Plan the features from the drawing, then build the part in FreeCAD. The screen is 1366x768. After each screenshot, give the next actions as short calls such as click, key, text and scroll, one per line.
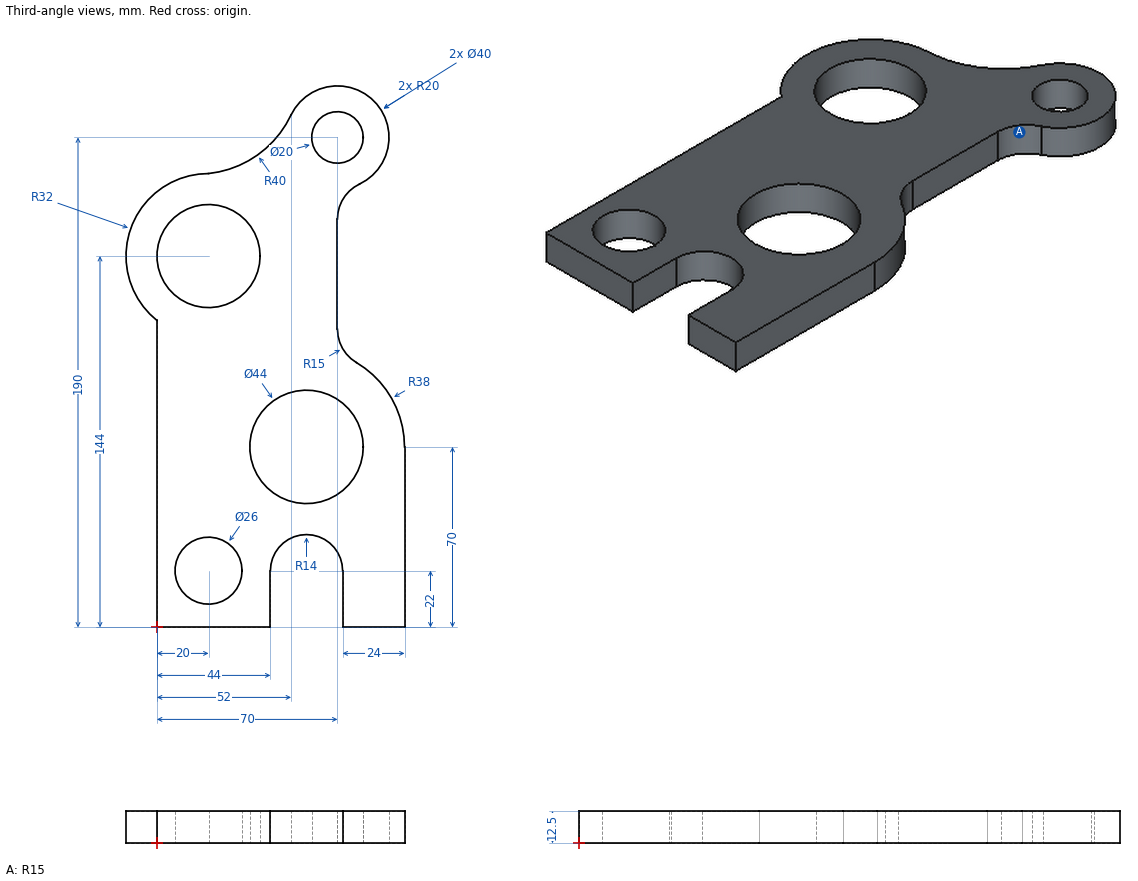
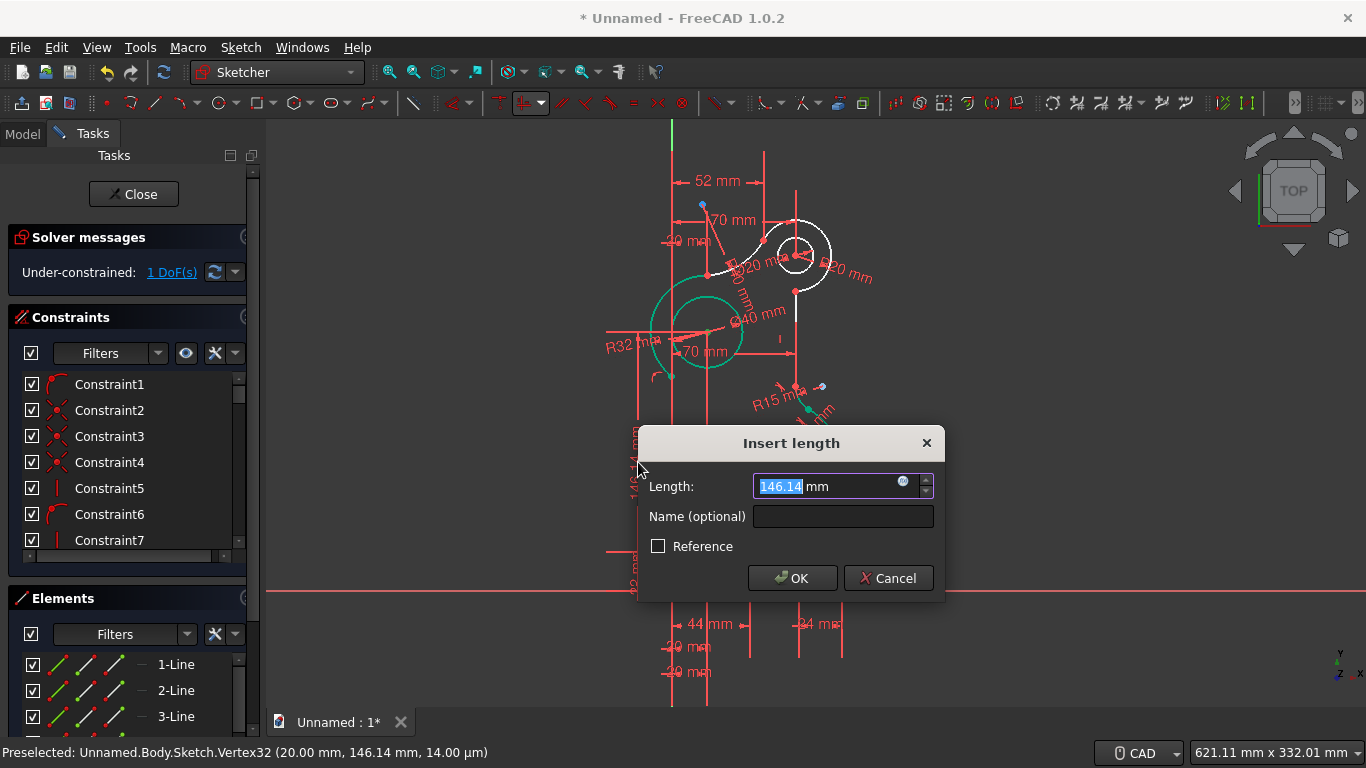
text(144)
key(Return)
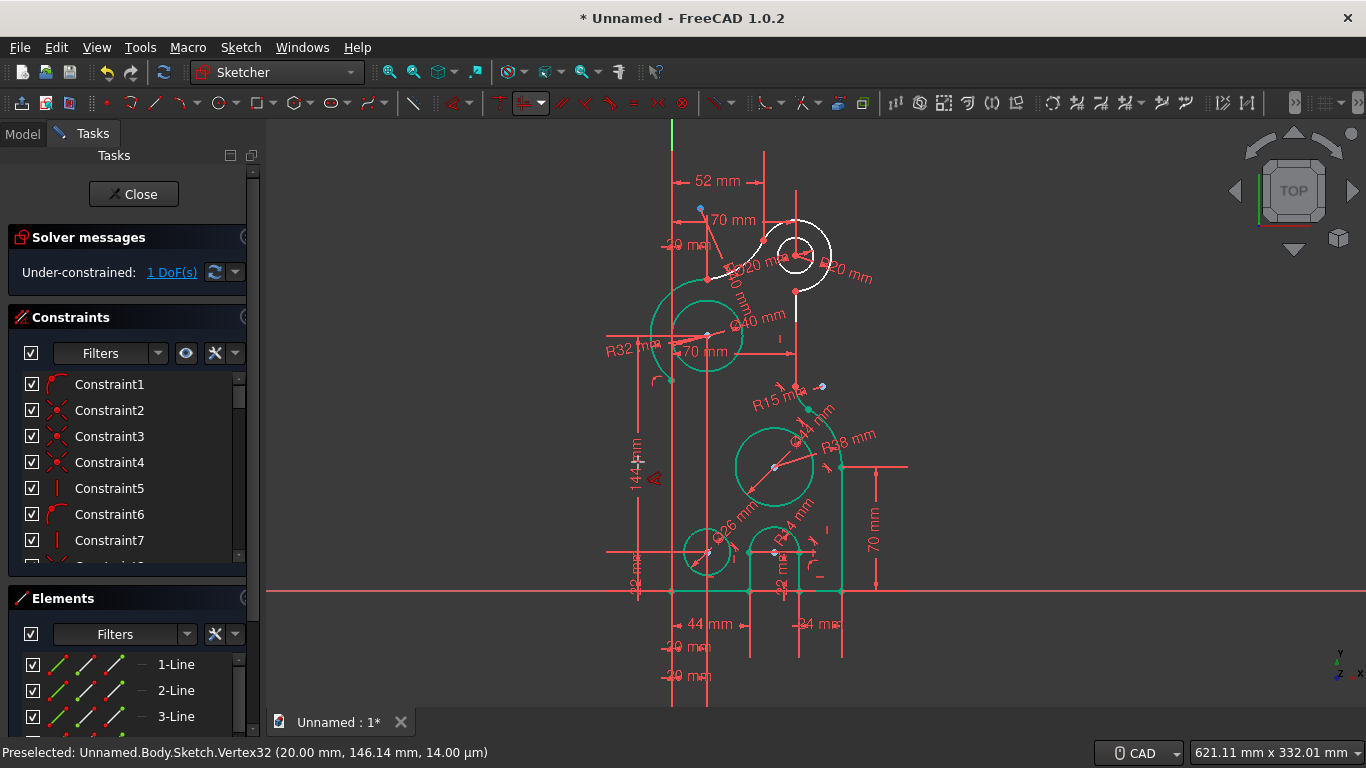
click(796, 256)
click(638, 423)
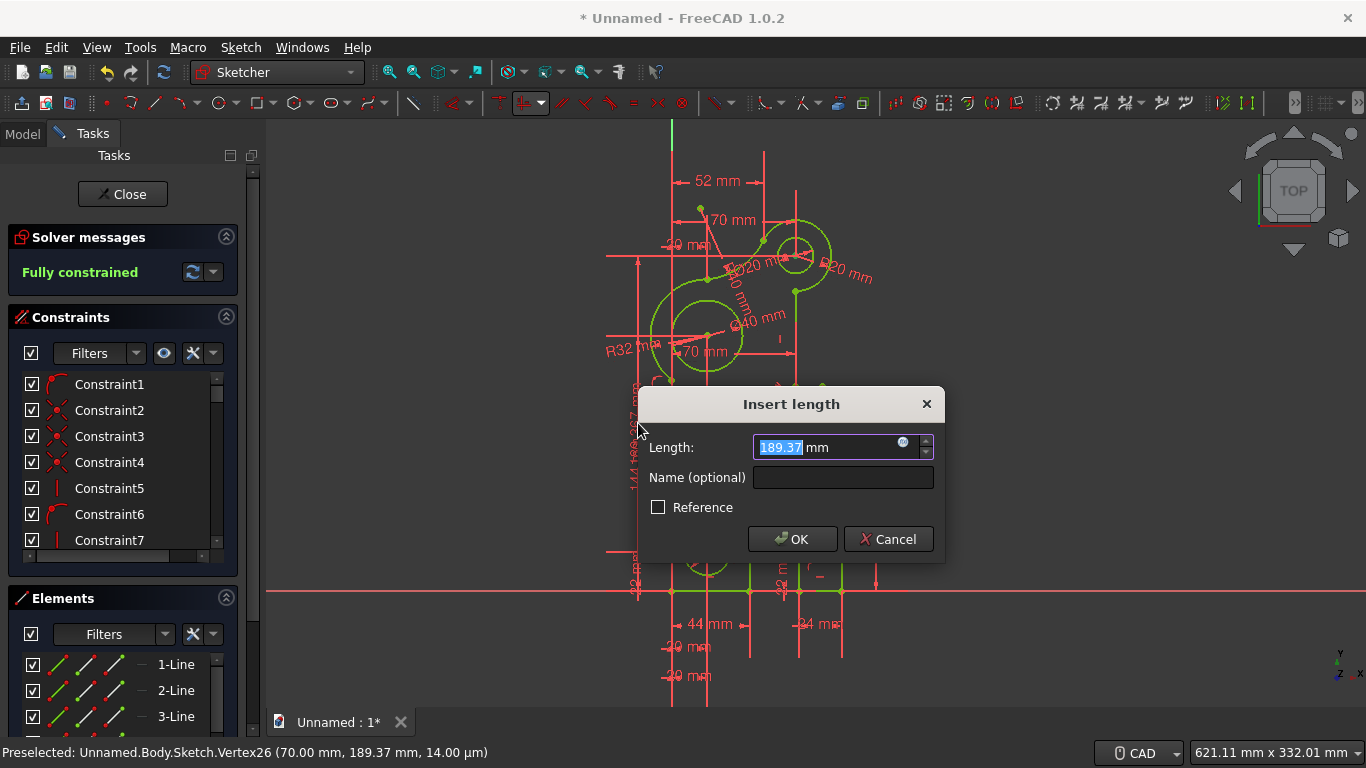
text(190)
key(Return)
key(Escape)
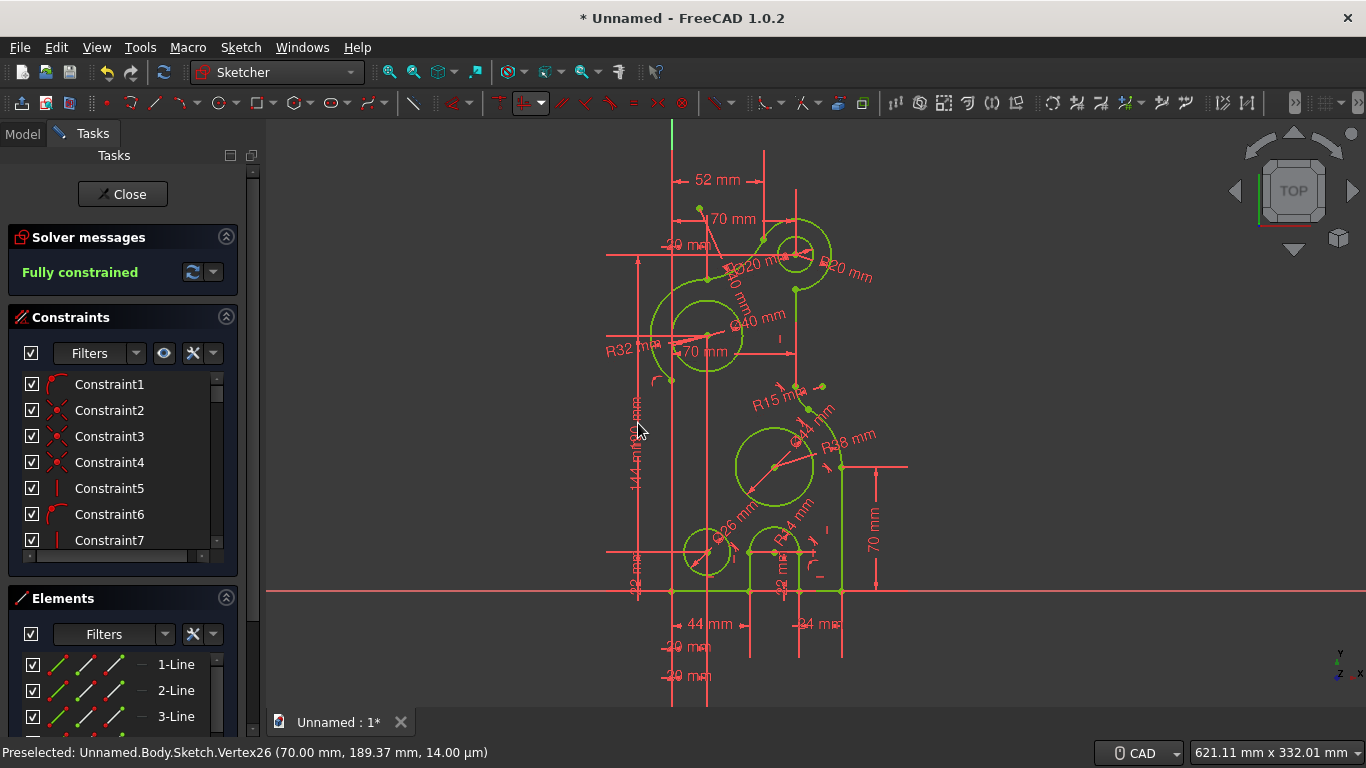
click(123, 194)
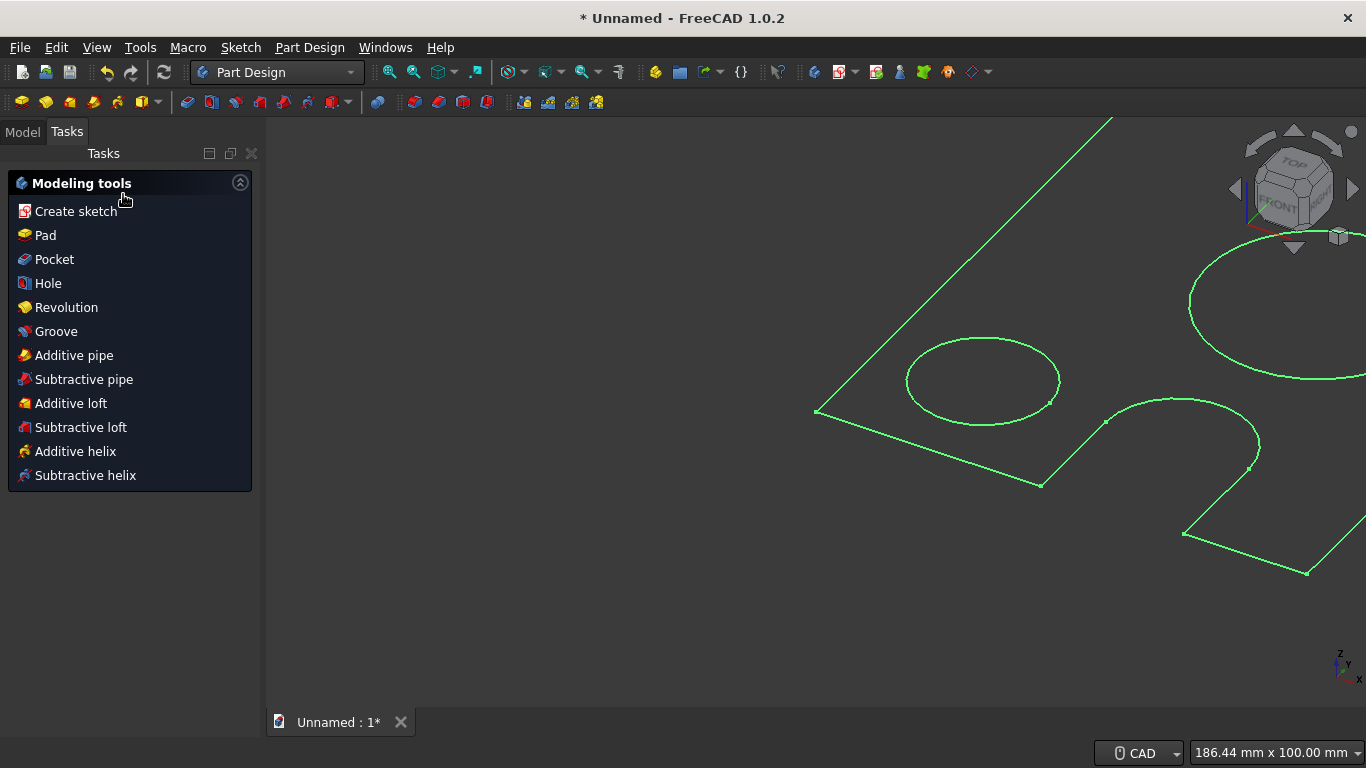
click(22, 102)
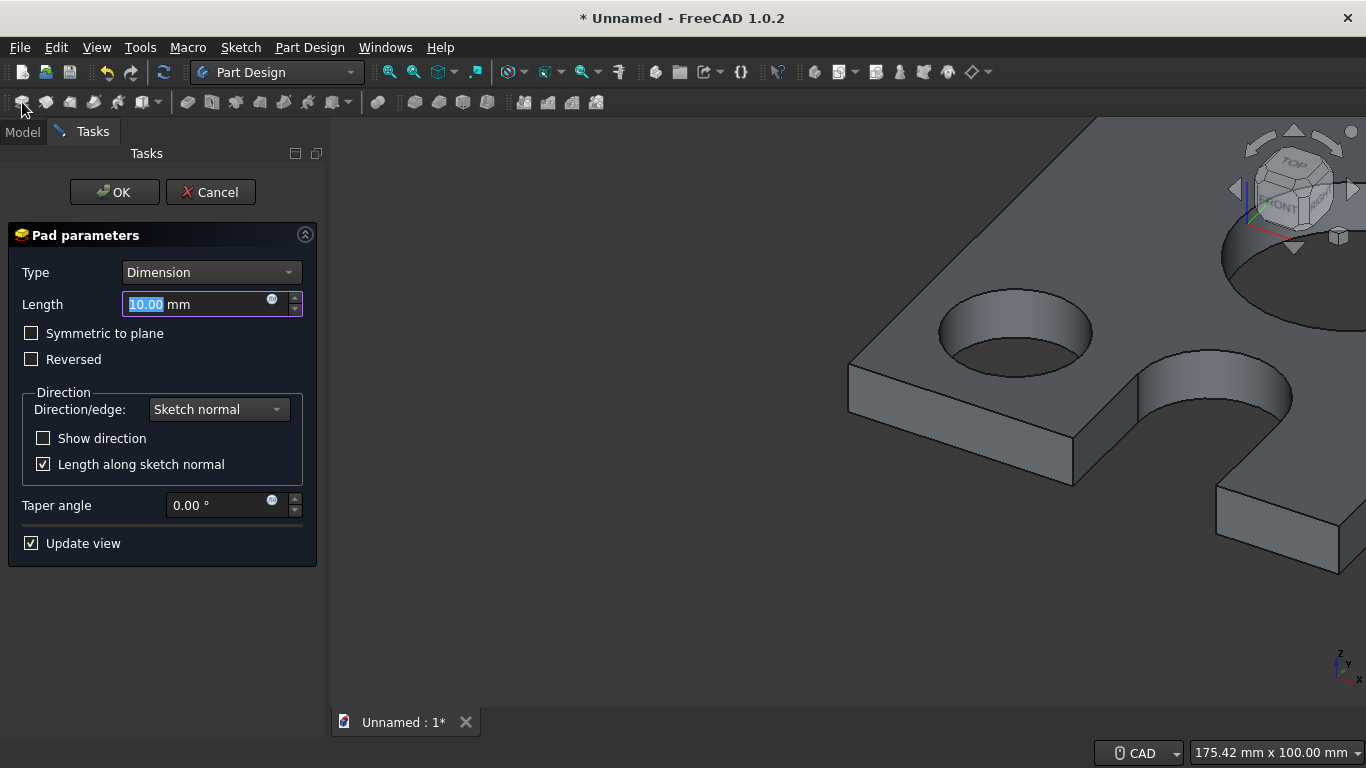
text(12.5)
key(Tab)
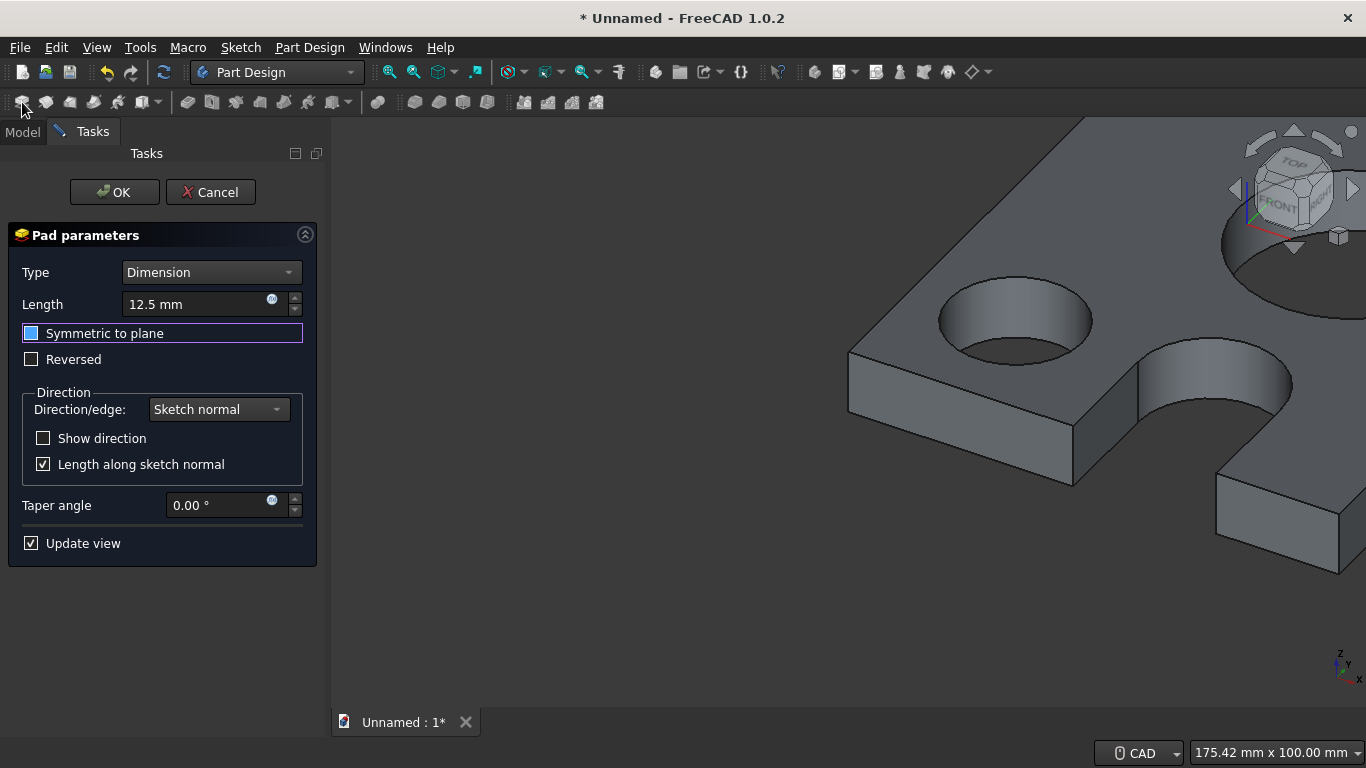
click(115, 192)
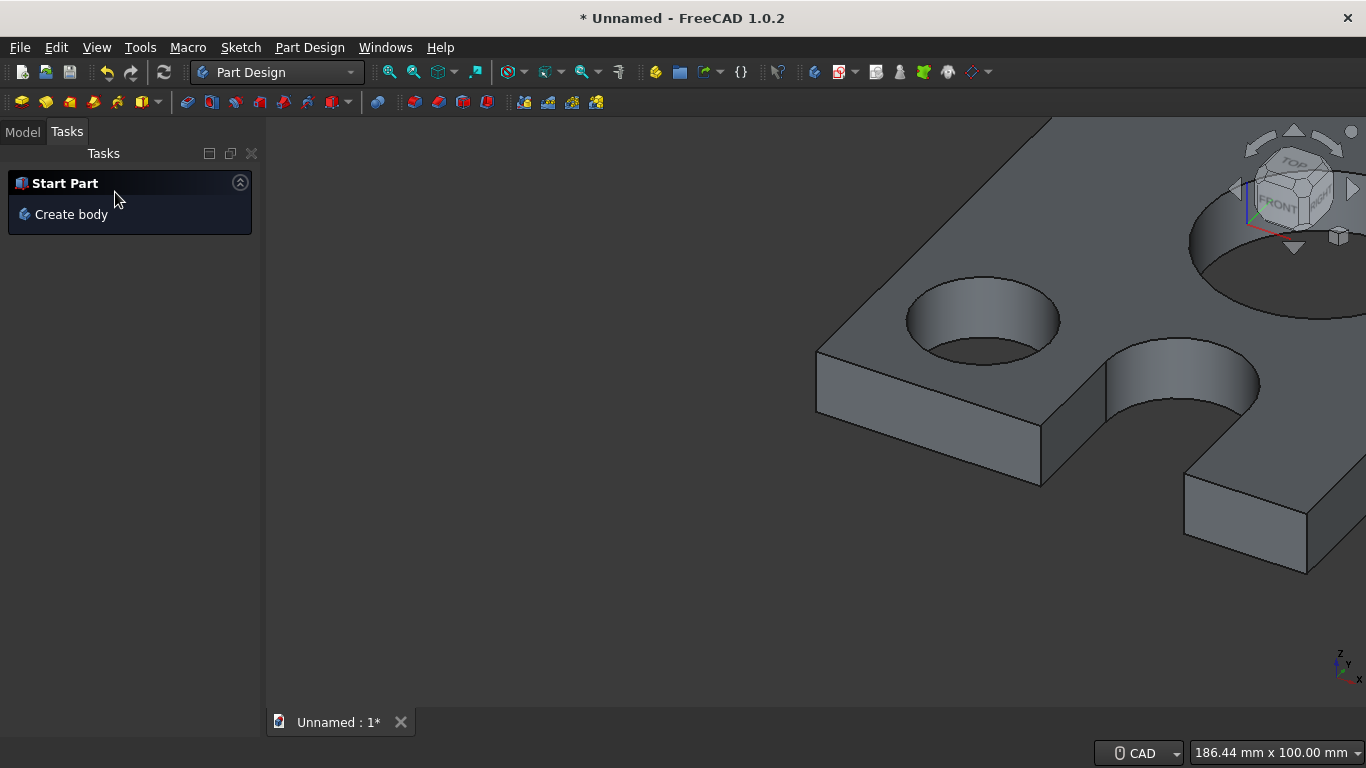
click(390, 72)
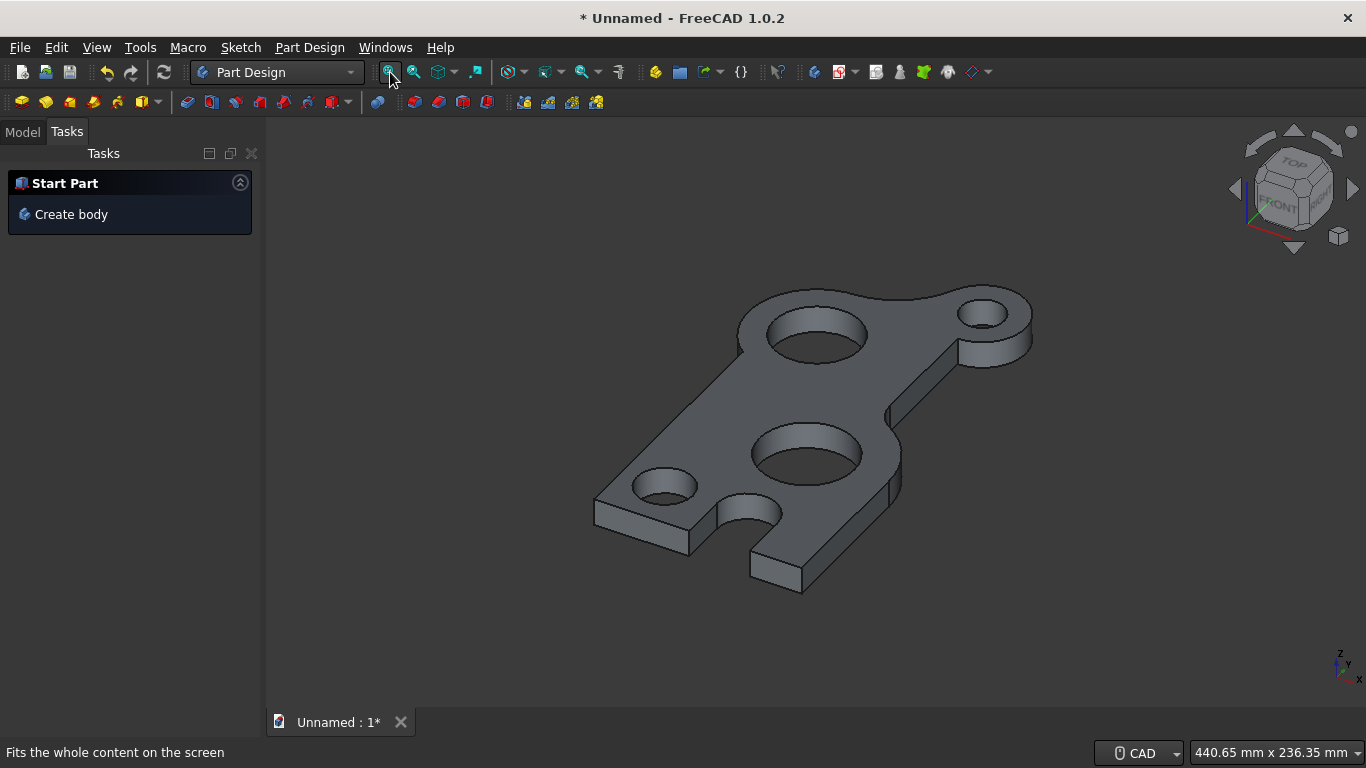
key(0)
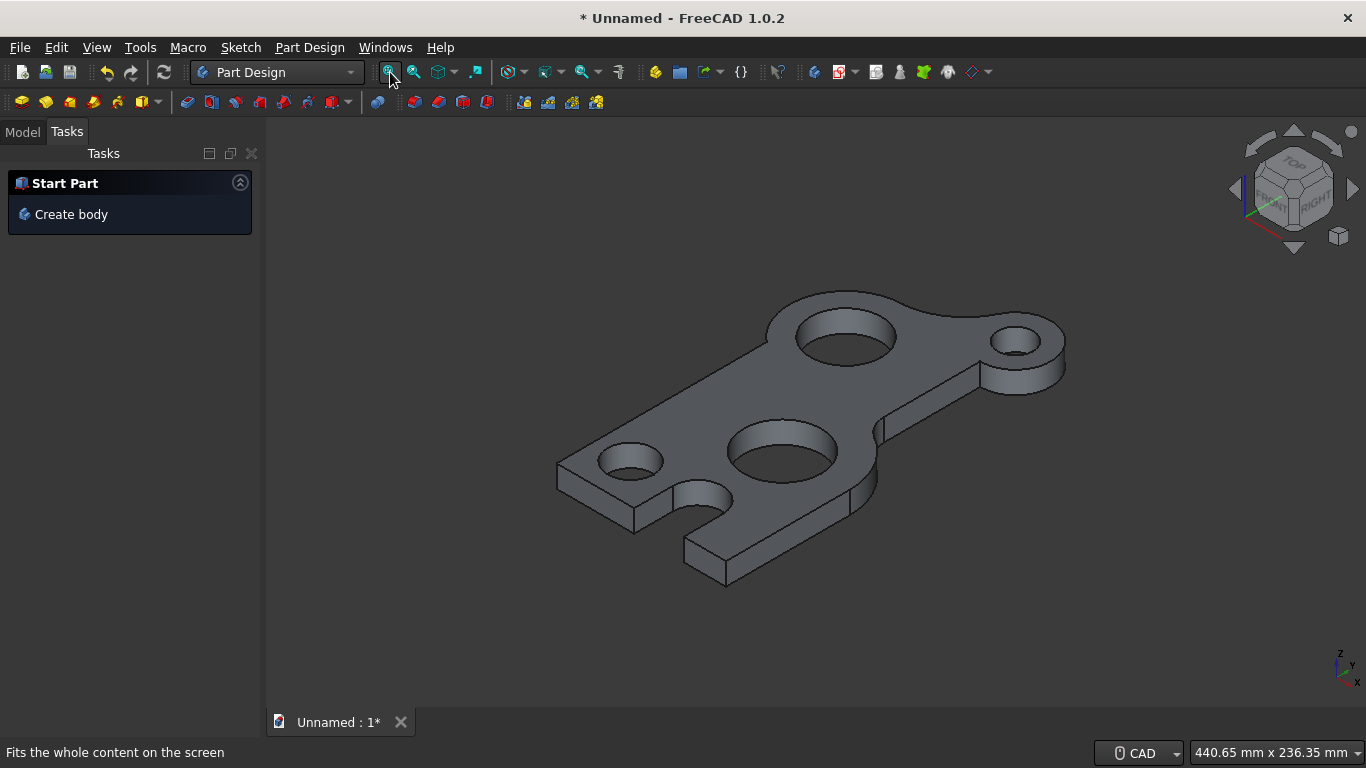
key(2)